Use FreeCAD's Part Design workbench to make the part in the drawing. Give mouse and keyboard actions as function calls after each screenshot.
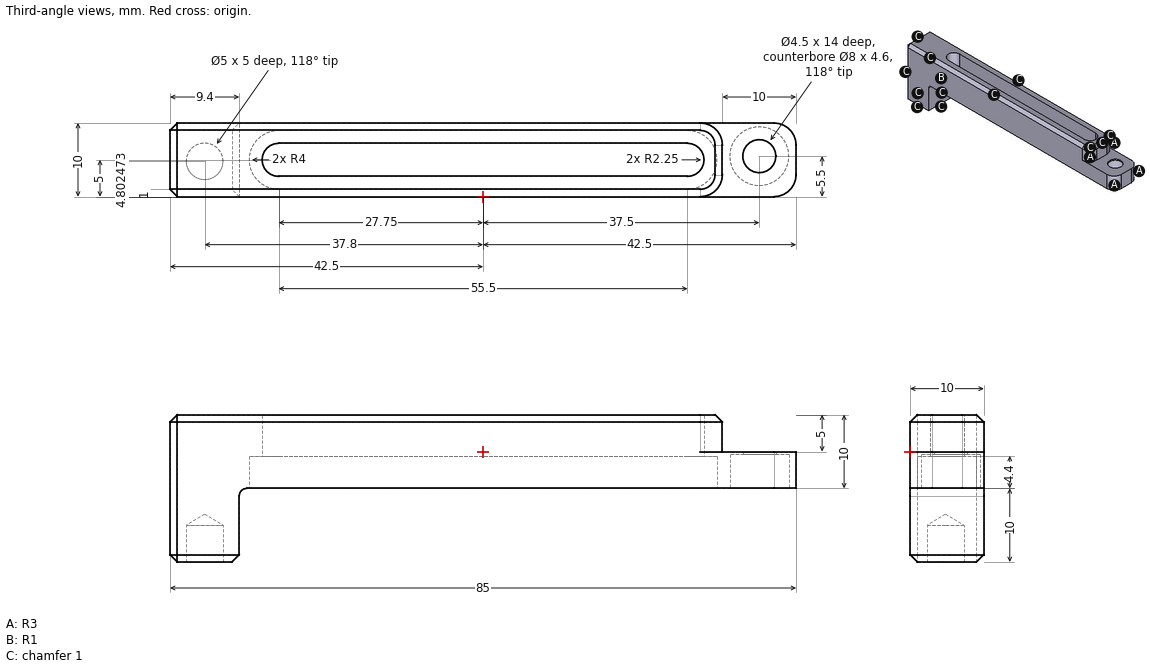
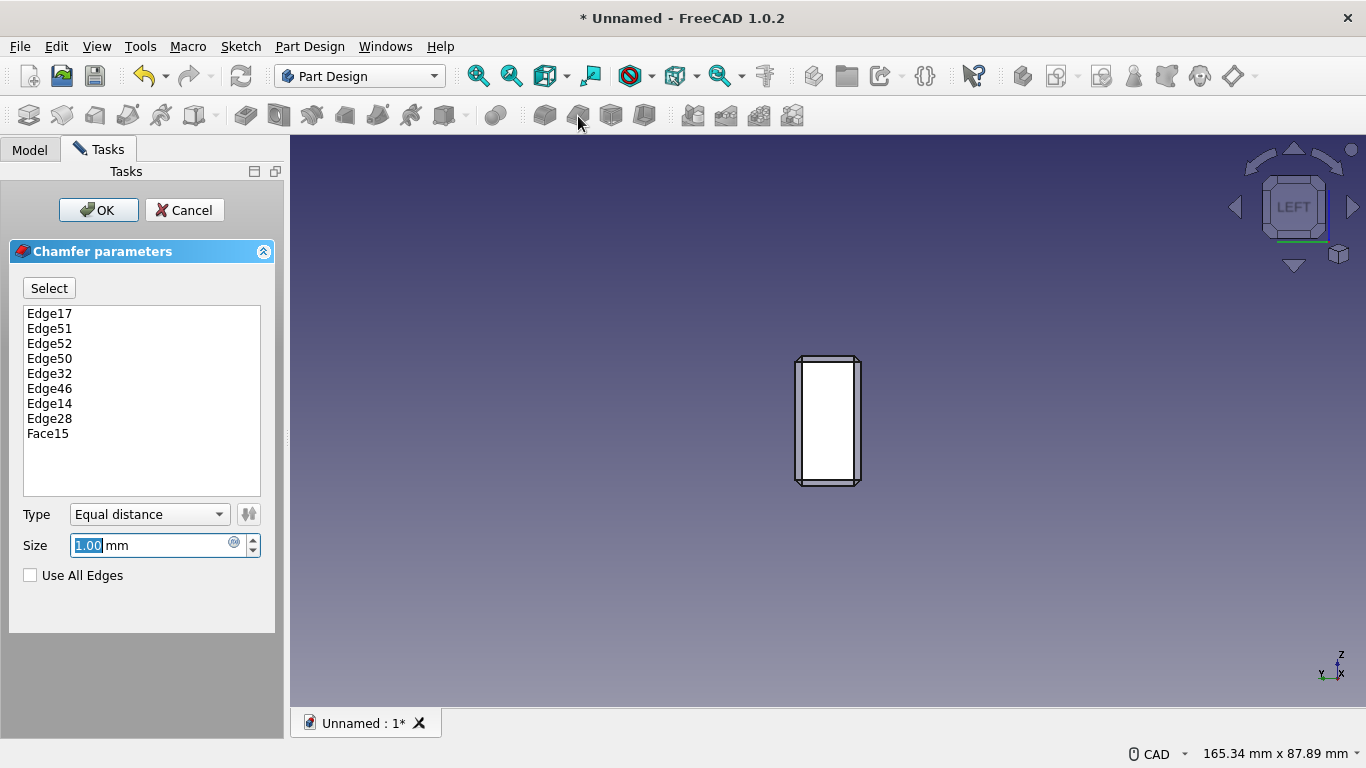
text(1)
key(Tab)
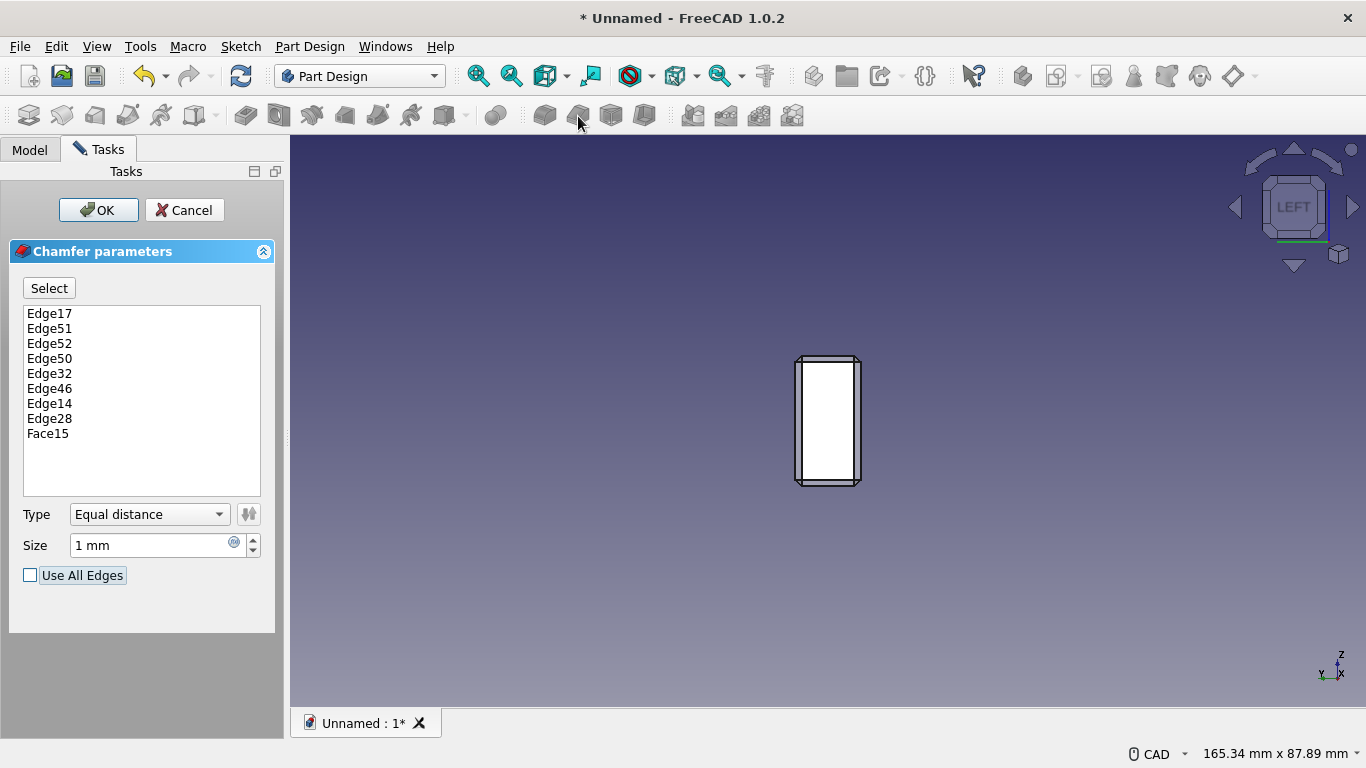
click(99, 210)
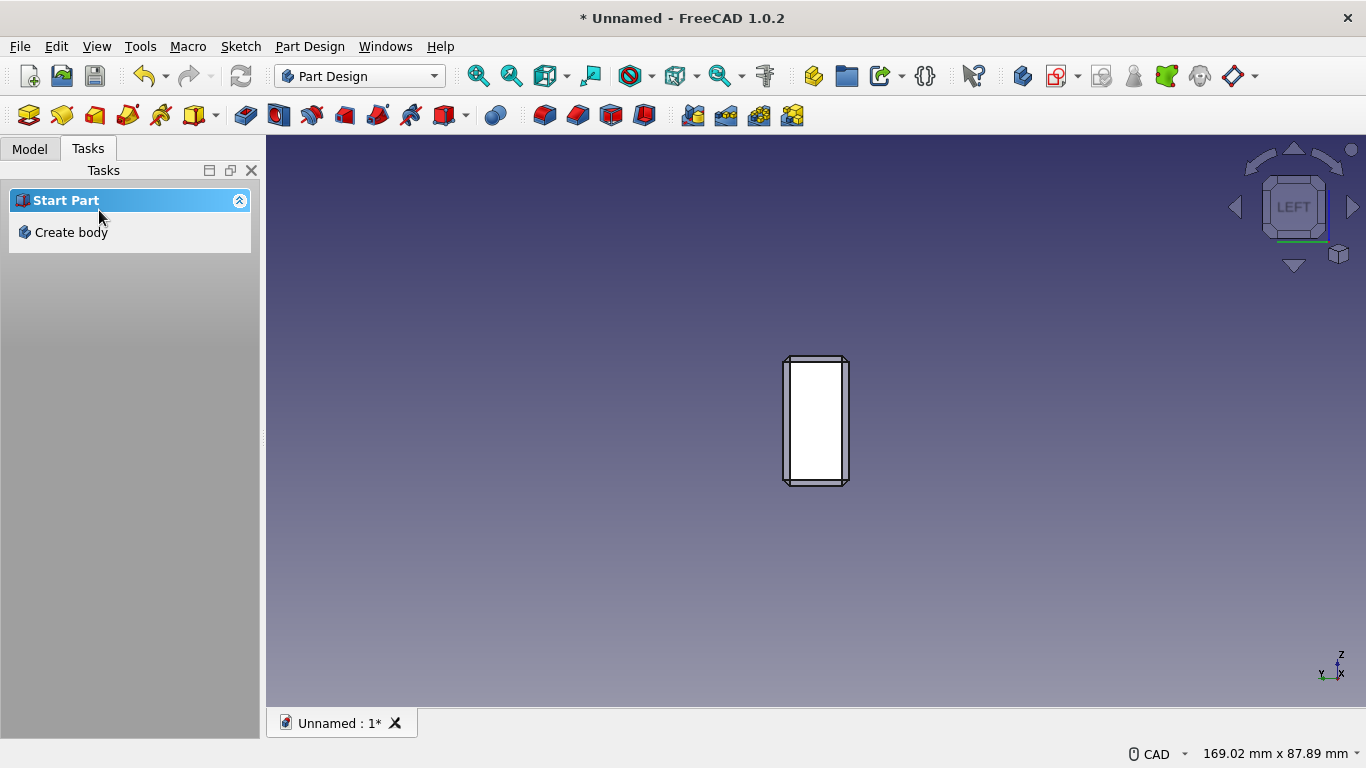
key(0)